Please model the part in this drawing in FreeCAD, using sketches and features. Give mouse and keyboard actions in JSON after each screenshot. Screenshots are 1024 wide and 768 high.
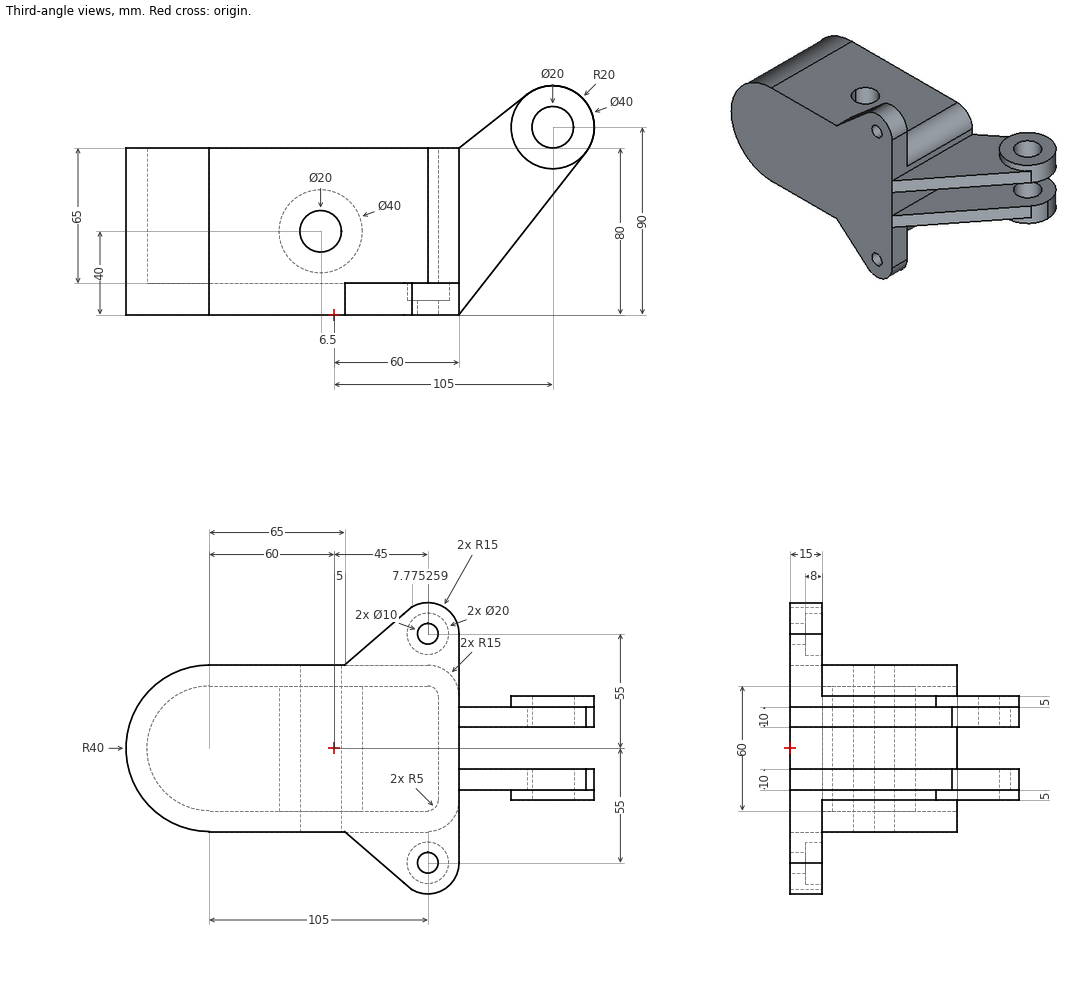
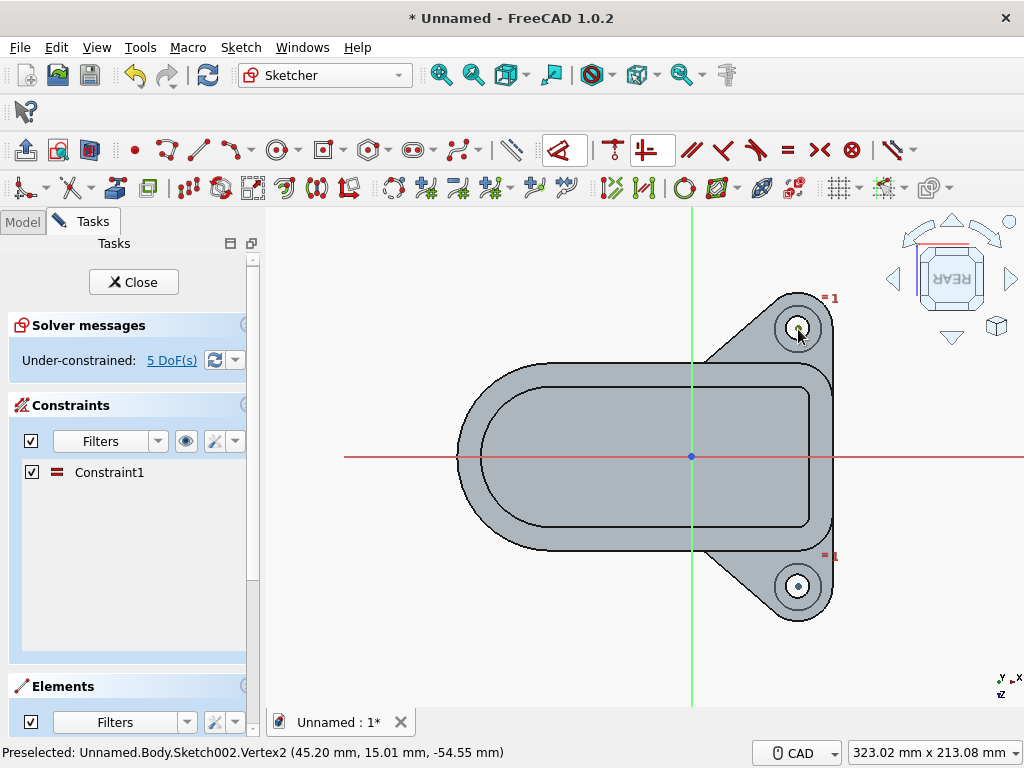
{"action": "left_click", "coordinate": [670, 150]}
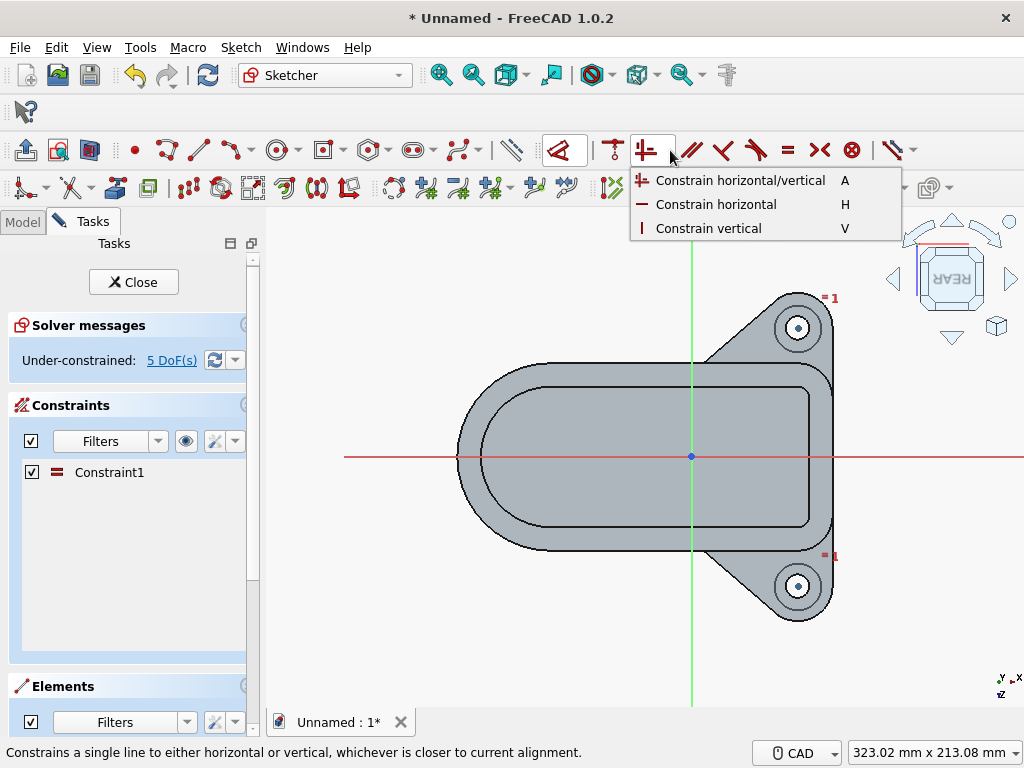
{"action": "left_click", "coordinate": [766, 228]}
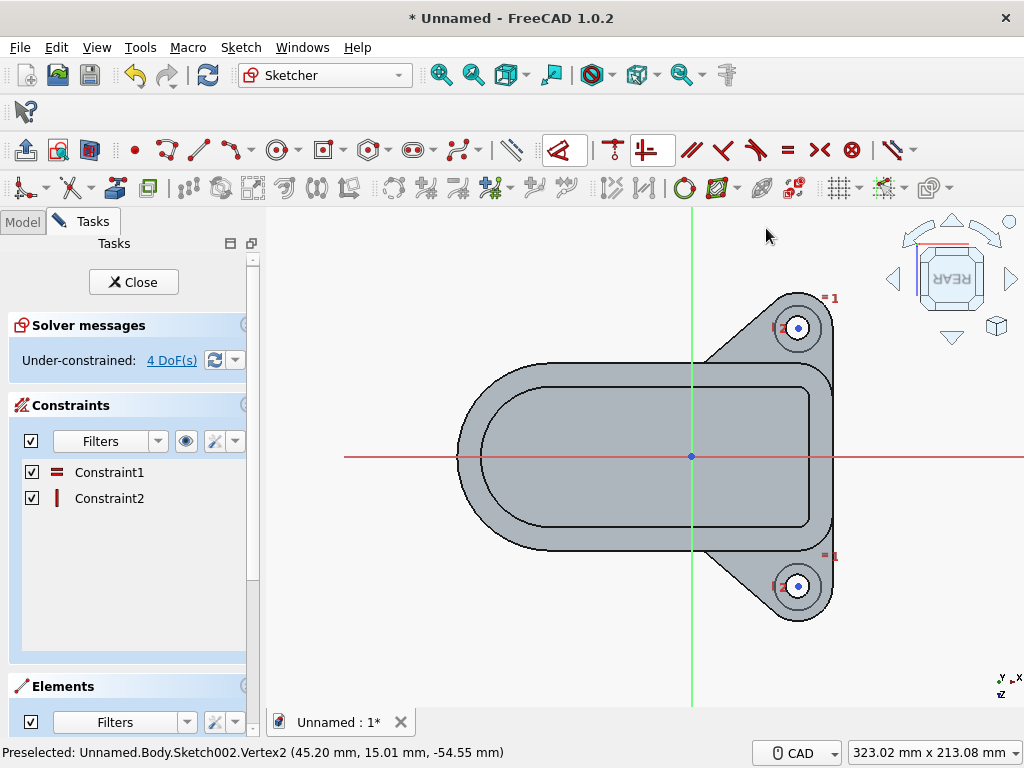
{"action": "left_click", "coordinate": [814, 570]}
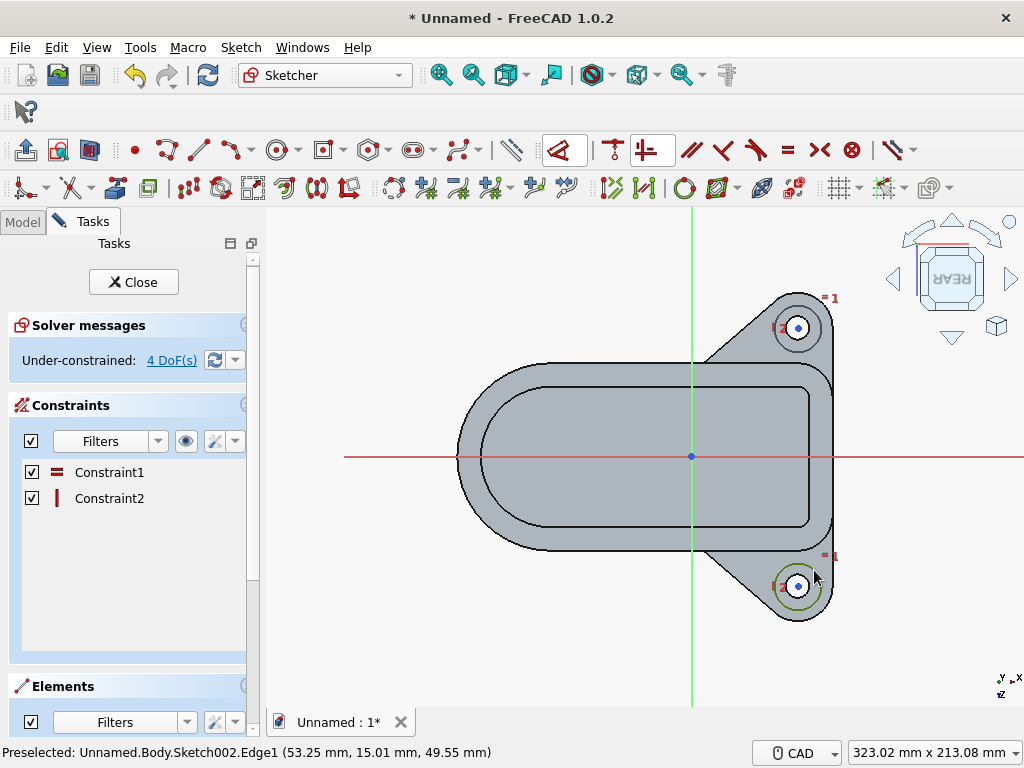
{"action": "left_click", "coordinate": [582, 150]}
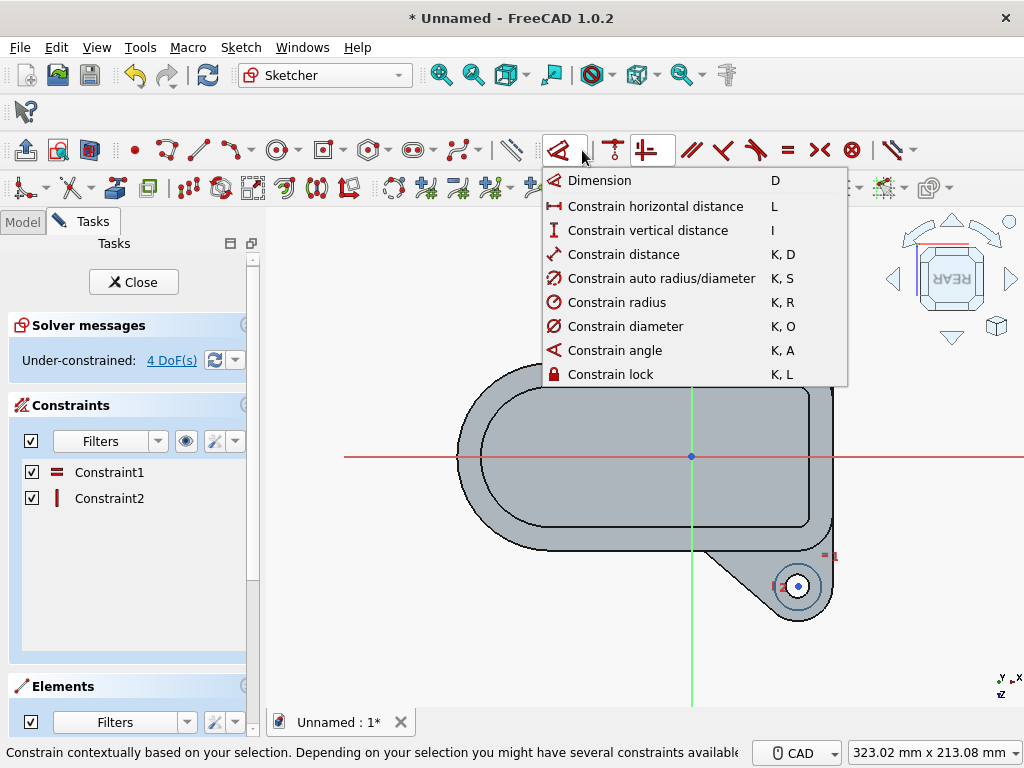
{"action": "left_click", "coordinate": [695, 326]}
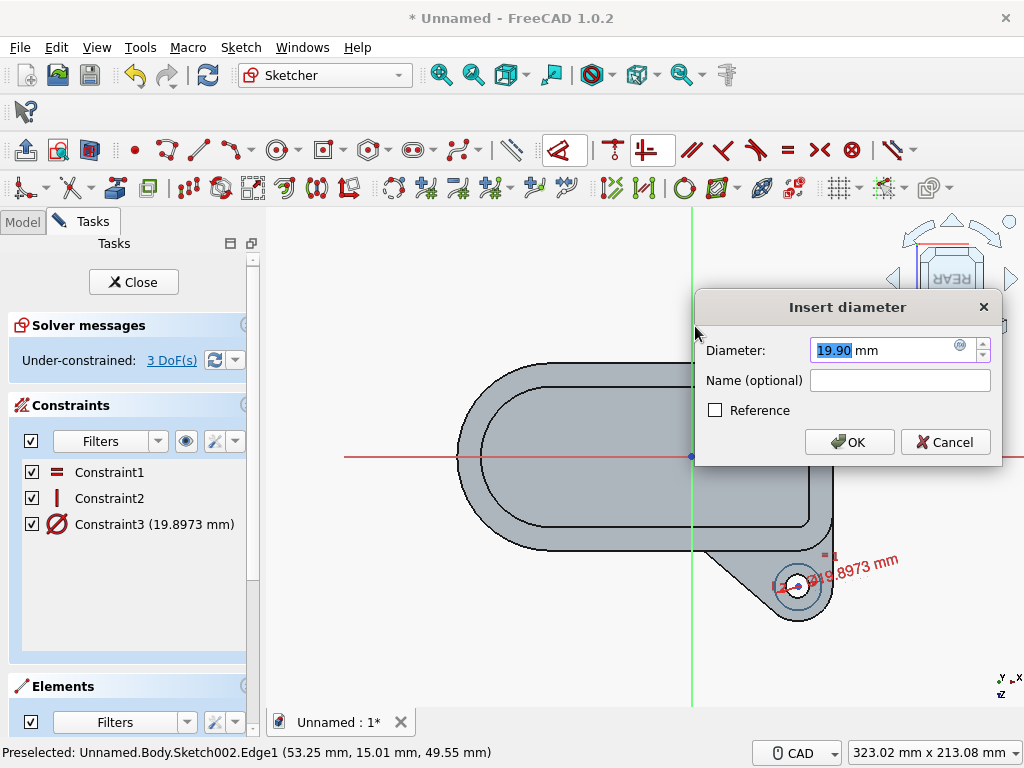
{"action": "type", "text": "20"}
{"action": "key", "text": "Return"}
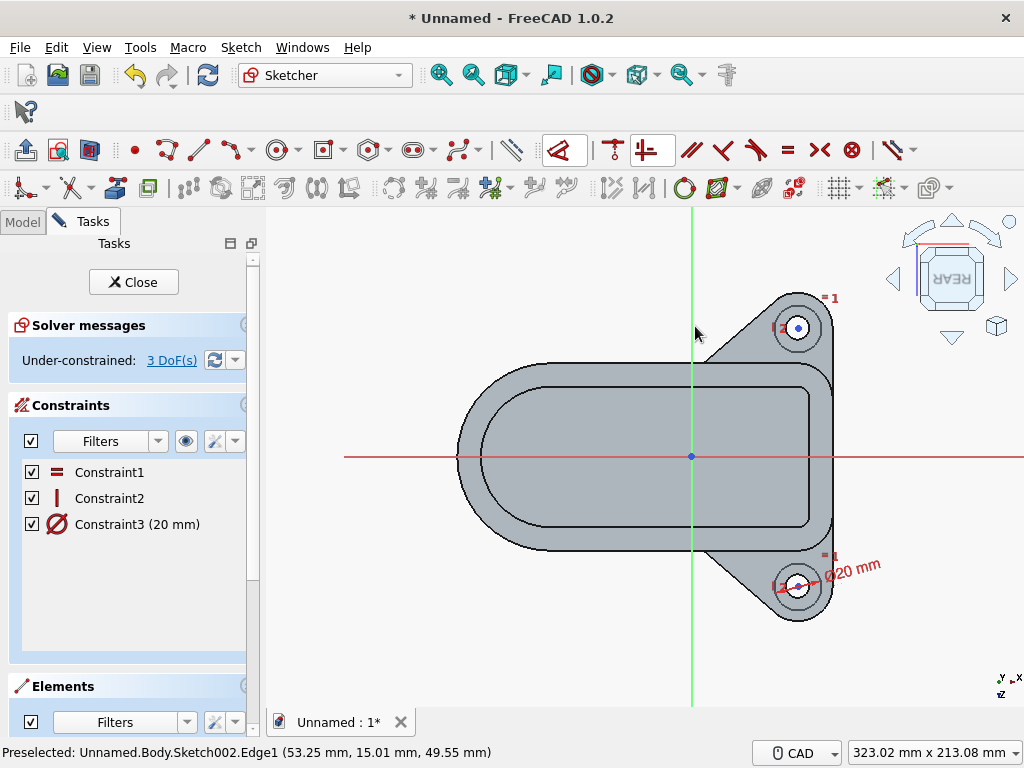
{"action": "left_click", "coordinate": [798, 587]}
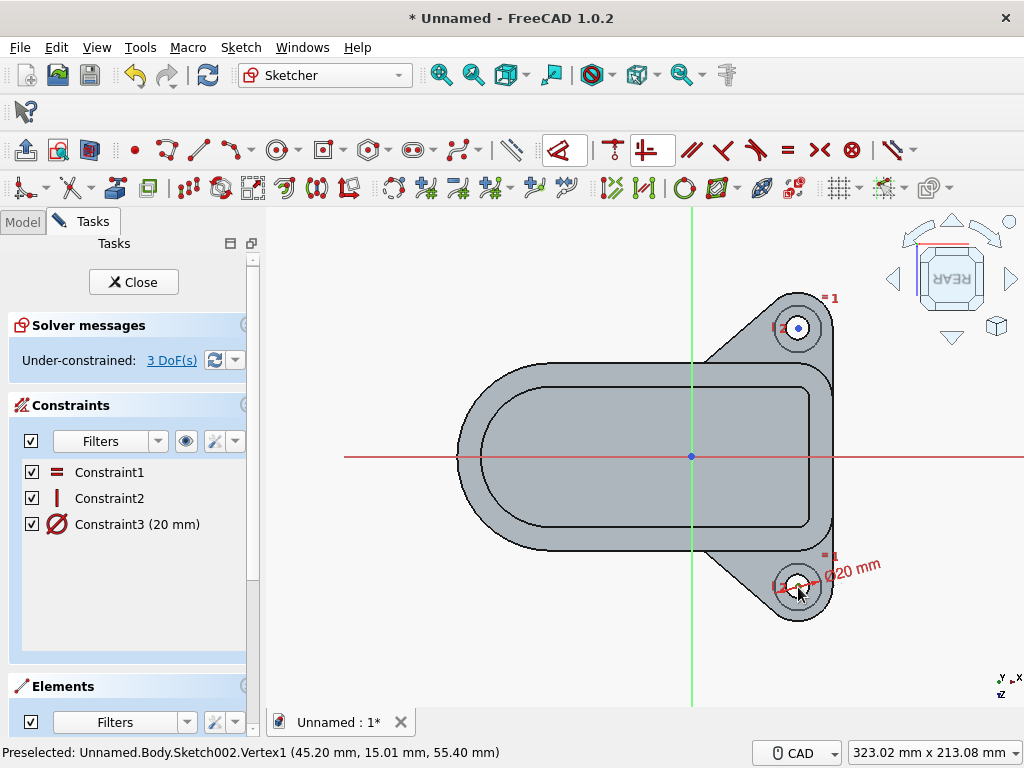
{"action": "left_click", "coordinate": [582, 150]}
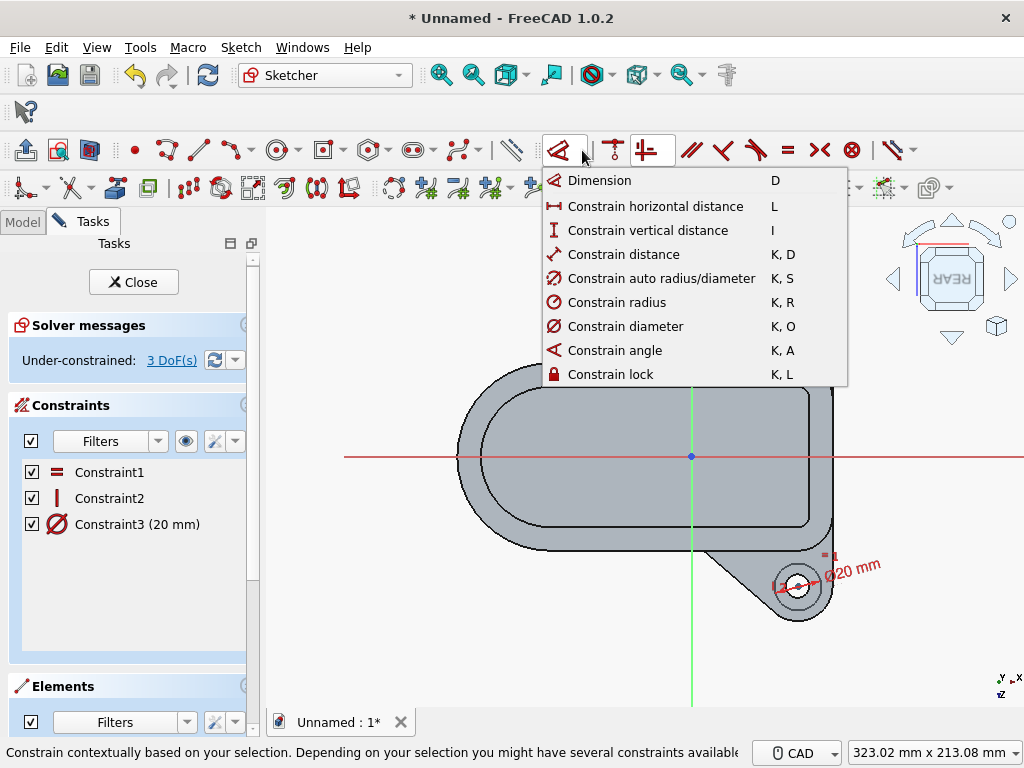
{"action": "left_click", "coordinate": [695, 206]}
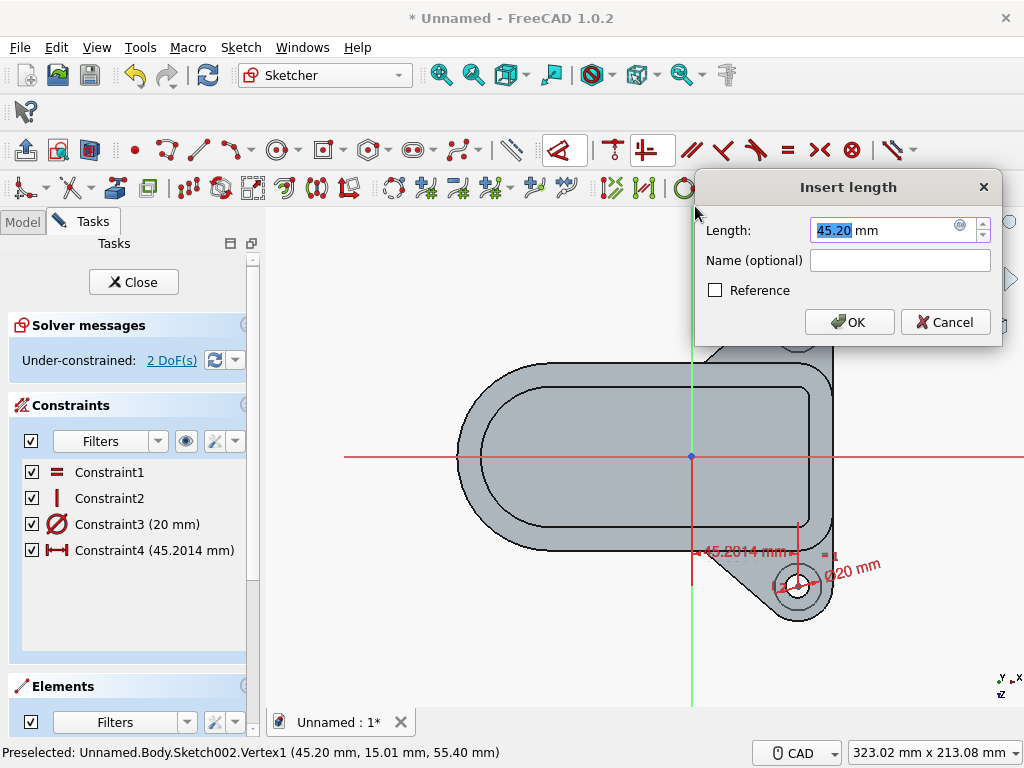
{"action": "type", "text": "45"}
{"action": "key", "text": "Return"}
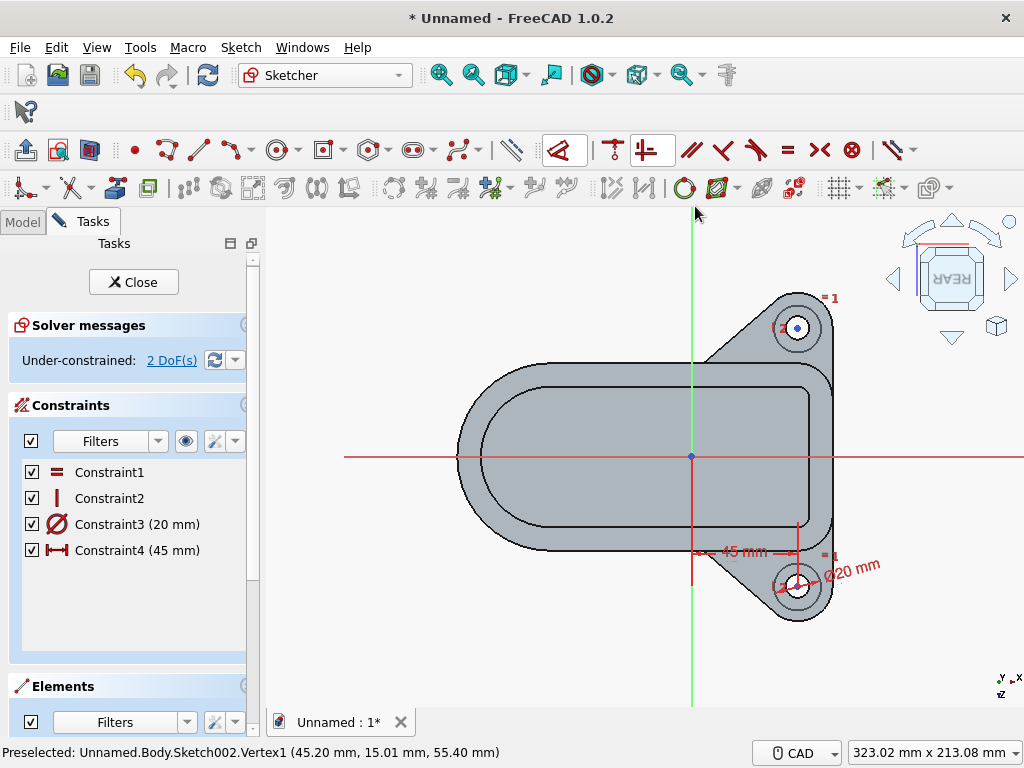
{"action": "left_click", "coordinate": [798, 587]}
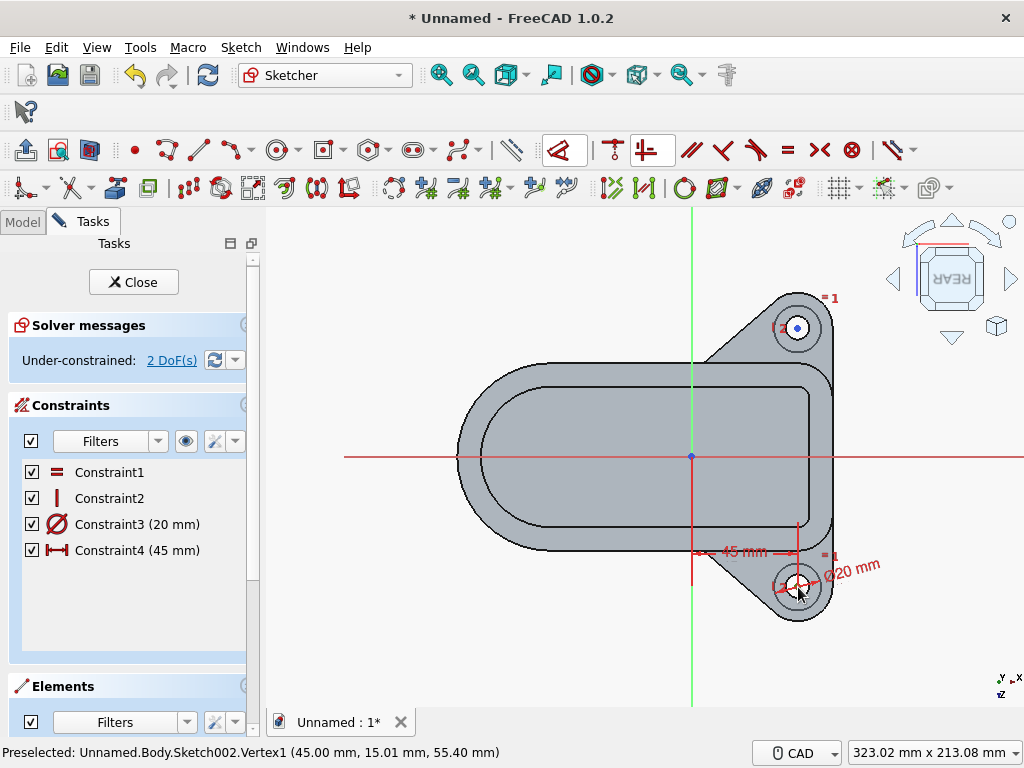
{"action": "key", "text": "i"}